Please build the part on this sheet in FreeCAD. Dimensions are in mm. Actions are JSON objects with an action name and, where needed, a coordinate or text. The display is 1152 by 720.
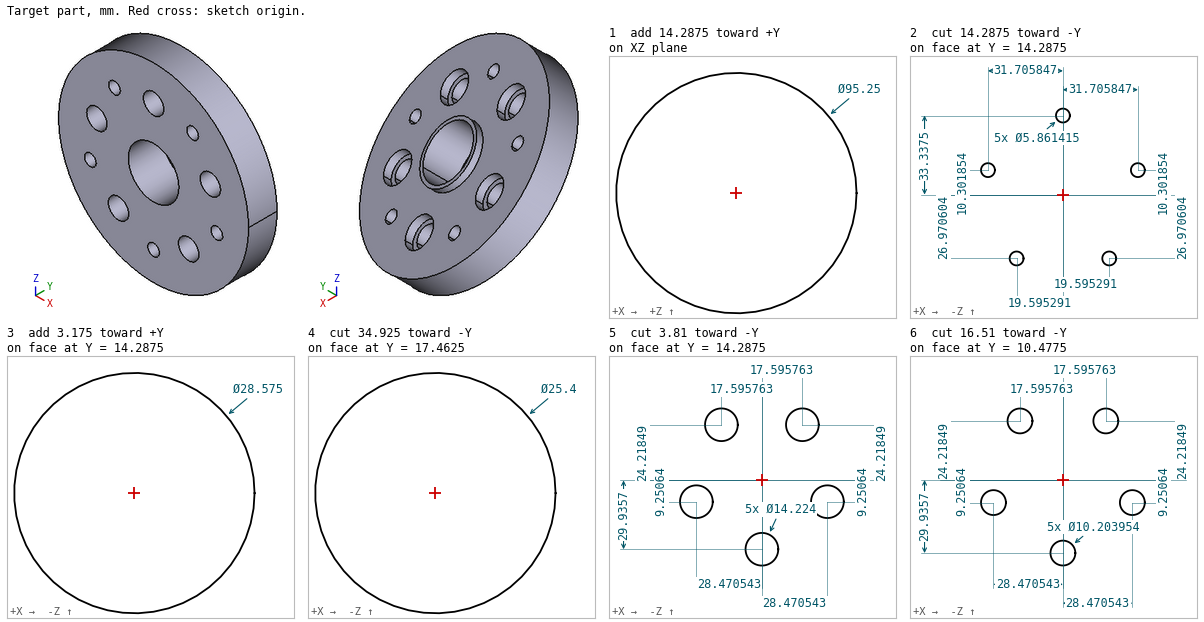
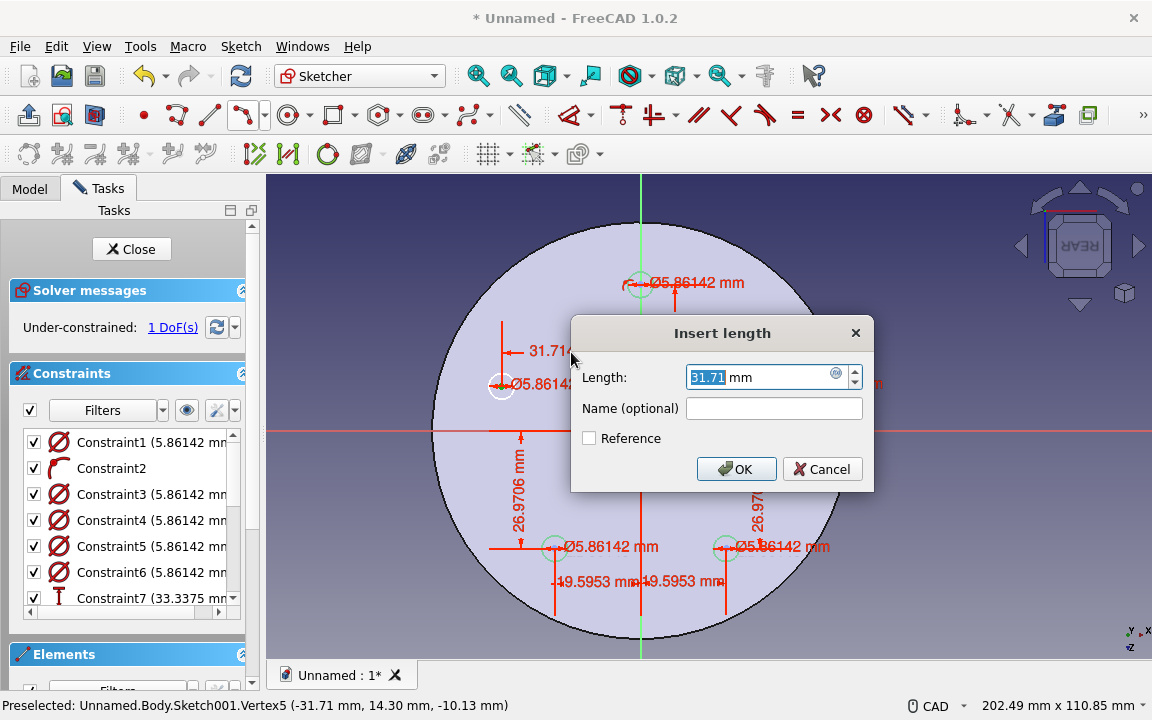
{"action": "type", "text": "31.705847"}
{"action": "key", "text": "Return"}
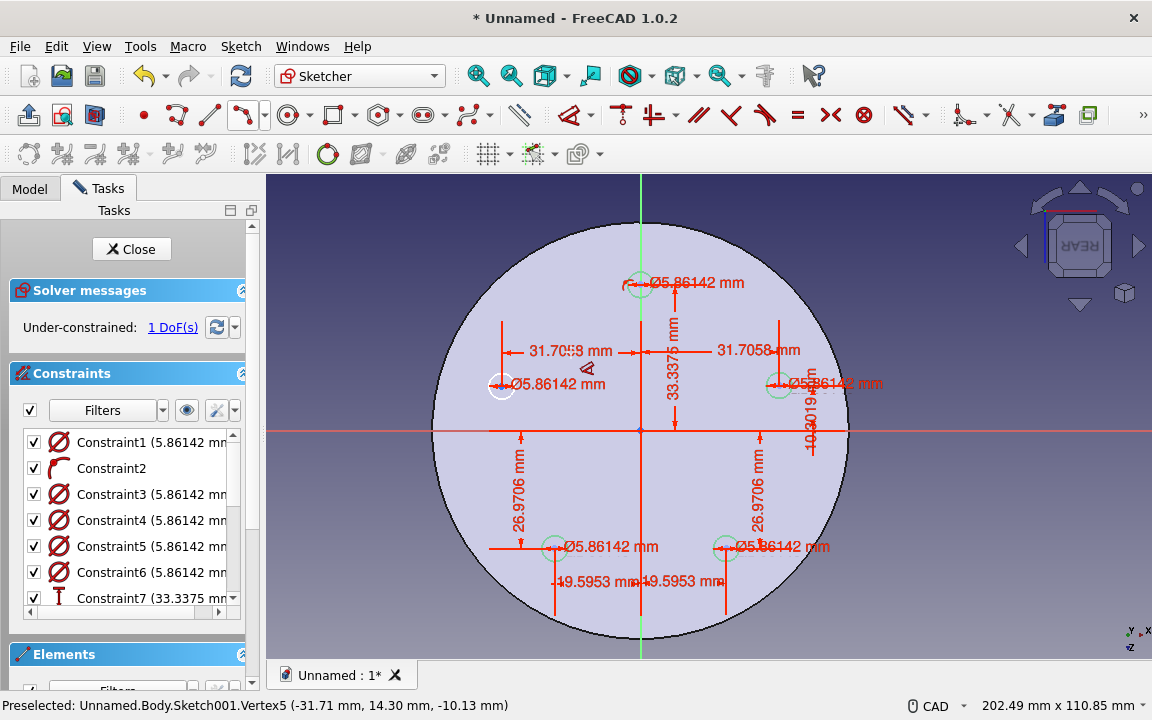
{"action": "left_click", "coordinate": [502, 386]}
{"action": "left_click", "coordinate": [468, 409]}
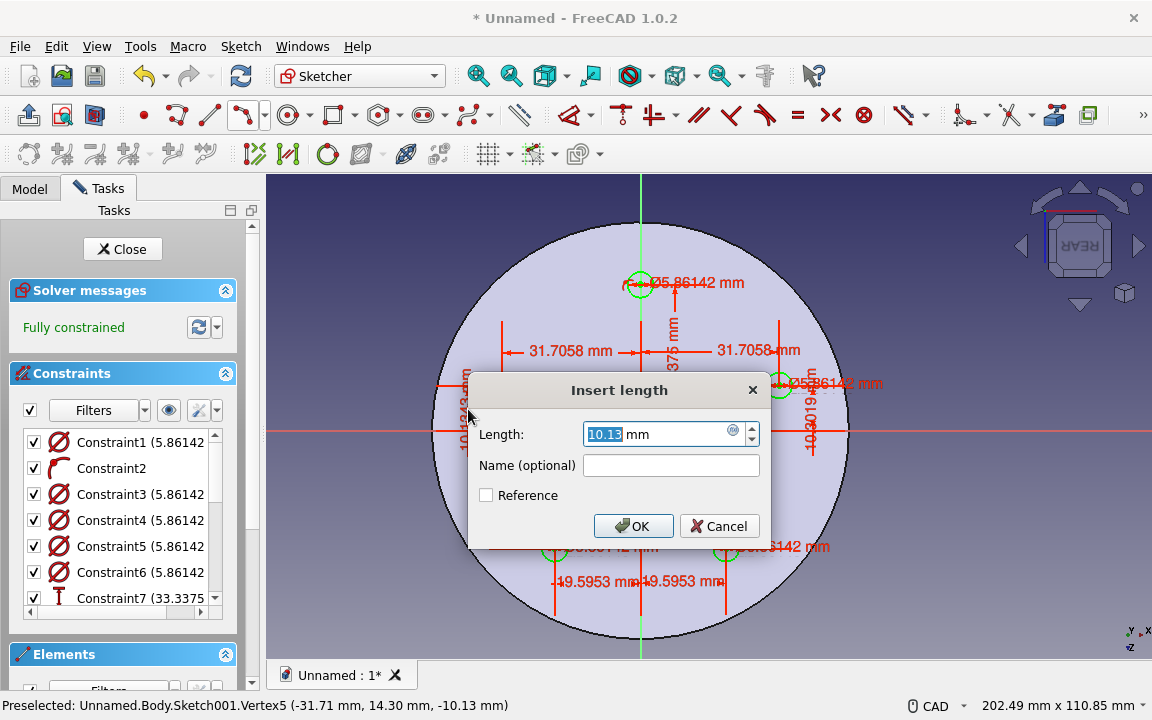
{"action": "type", "text": "10.301854"}
{"action": "key", "text": "Return"}
{"action": "key", "text": "Escape"}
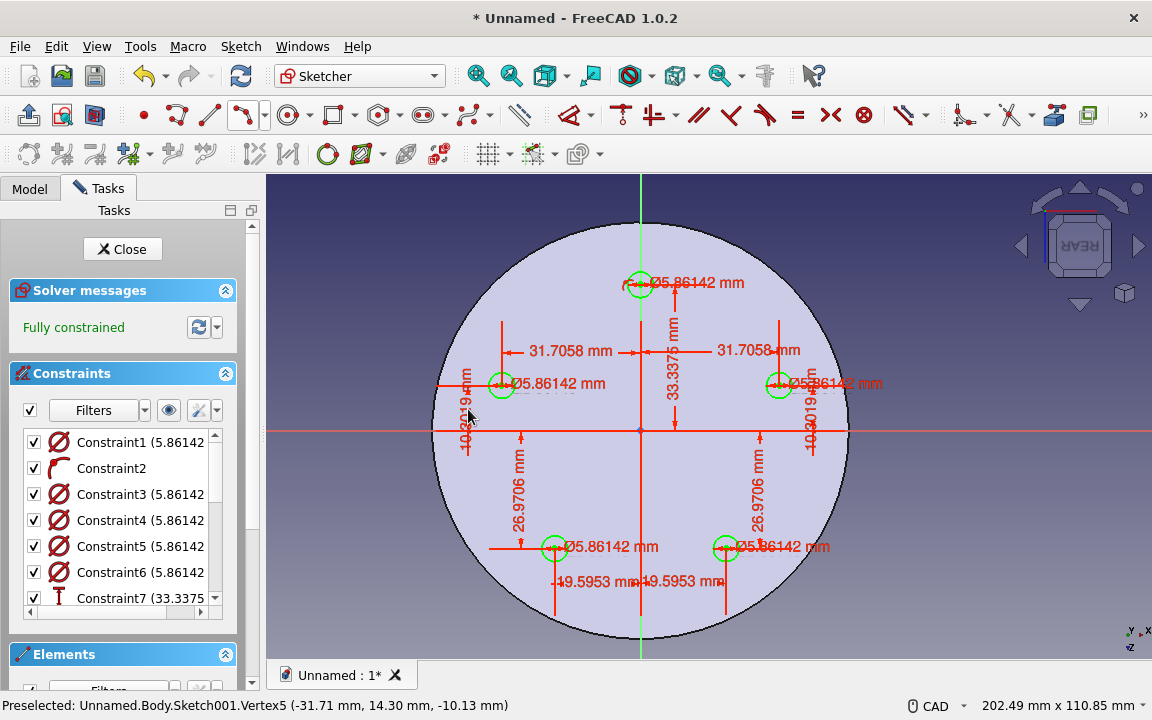
{"action": "left_click", "coordinate": [123, 249]}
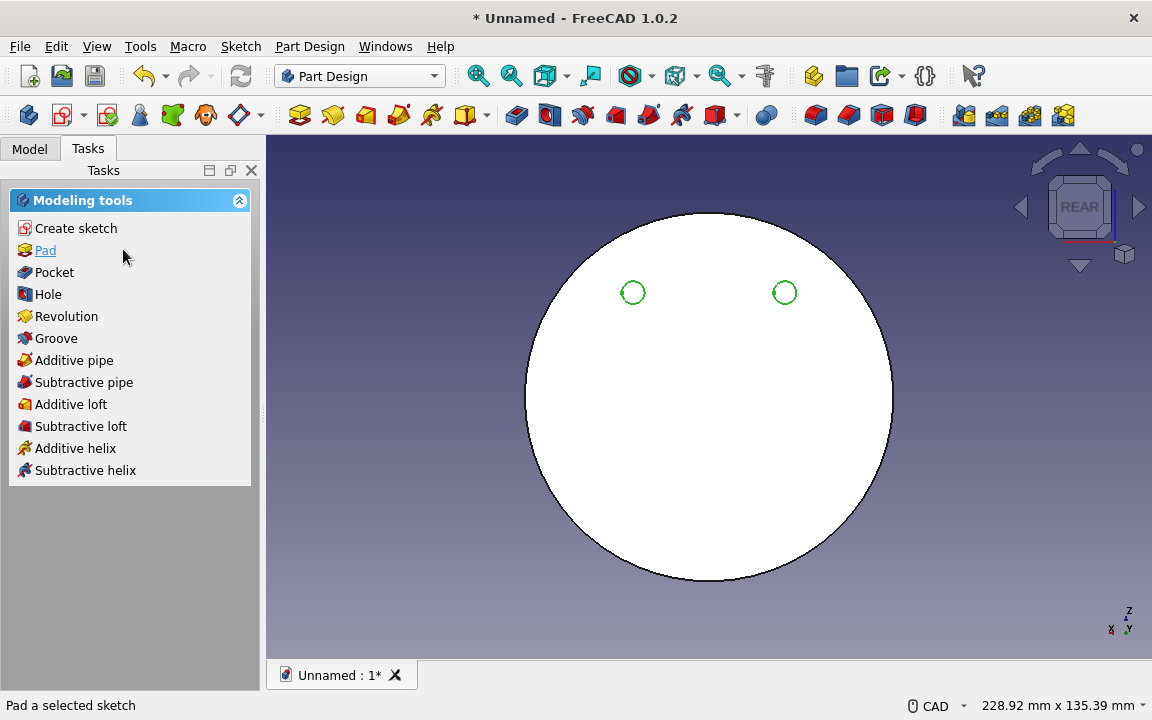
{"action": "left_click", "coordinate": [517, 116]}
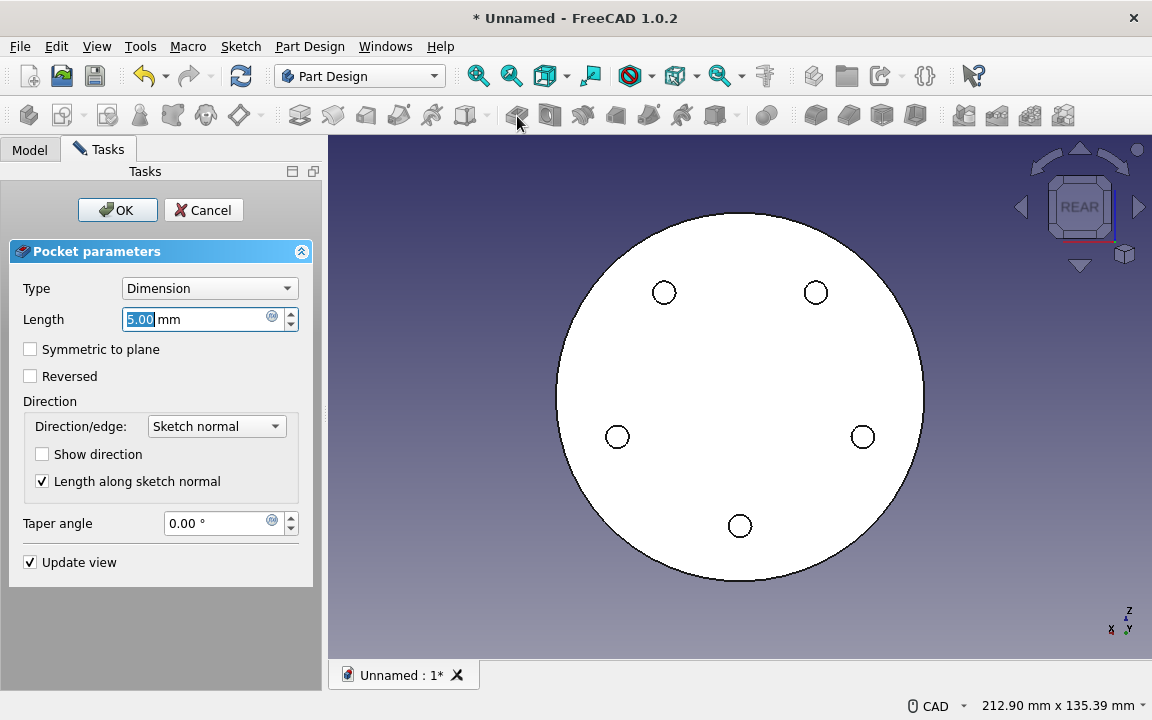
{"action": "type", "text": "14.2875"}
{"action": "key", "text": "Tab"}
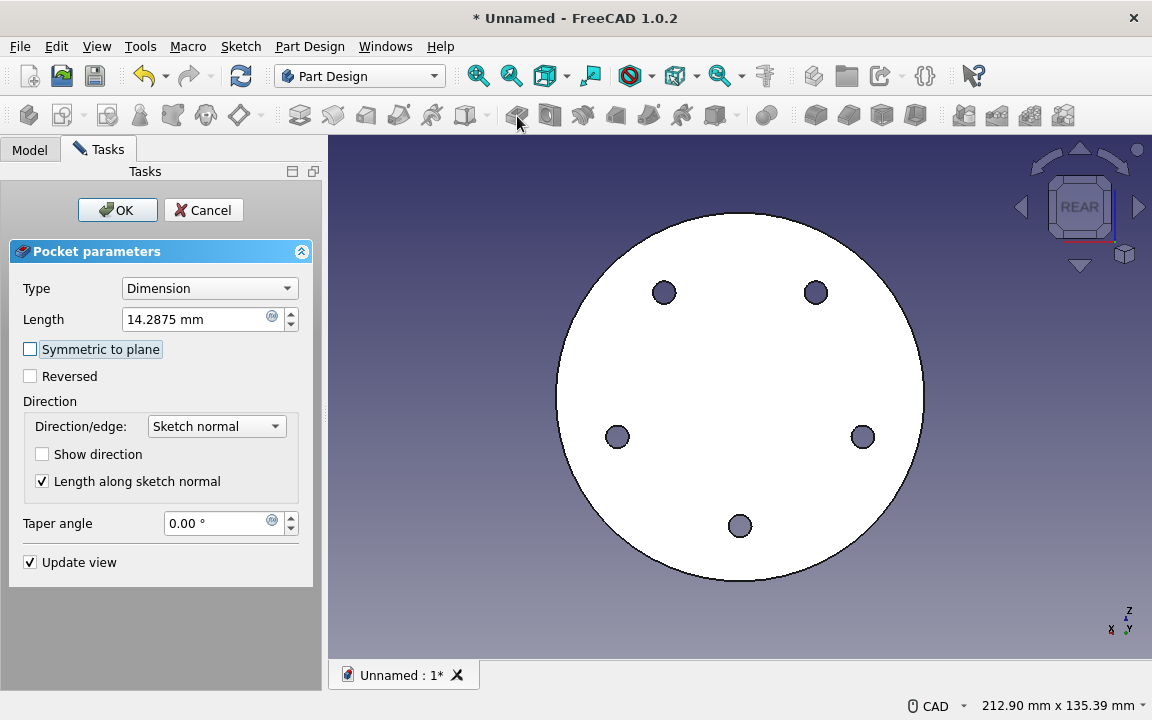
{"action": "left_click", "coordinate": [118, 210]}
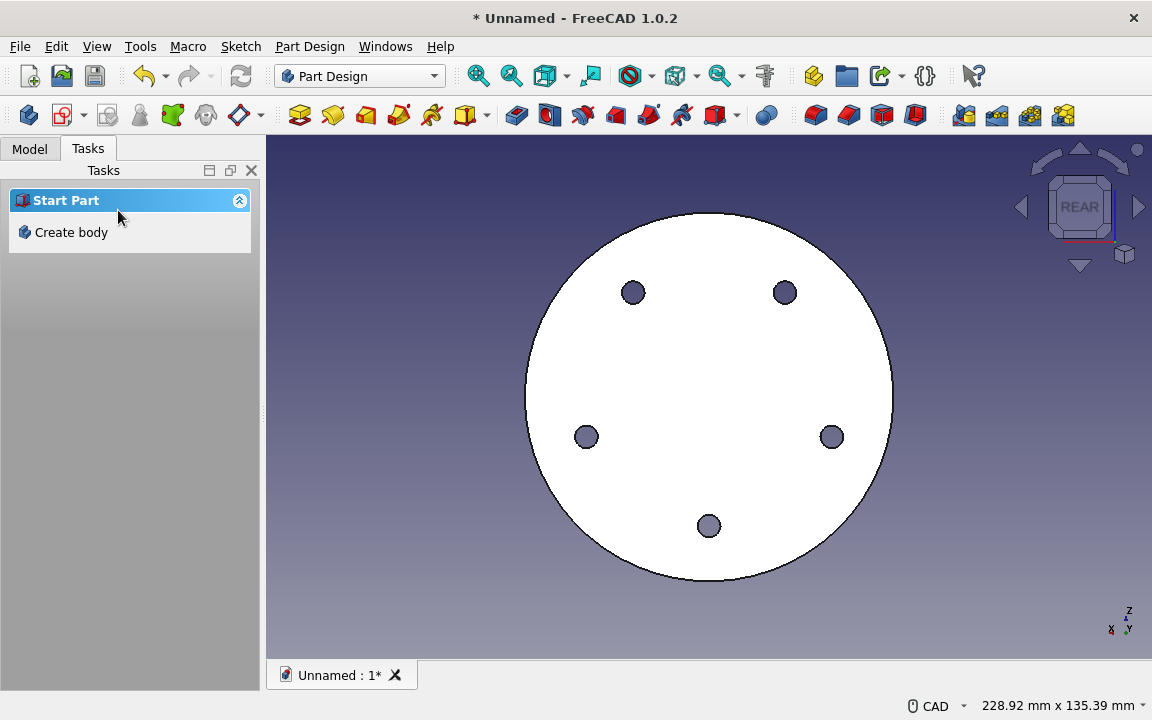
{"action": "left_click", "coordinate": [709, 396]}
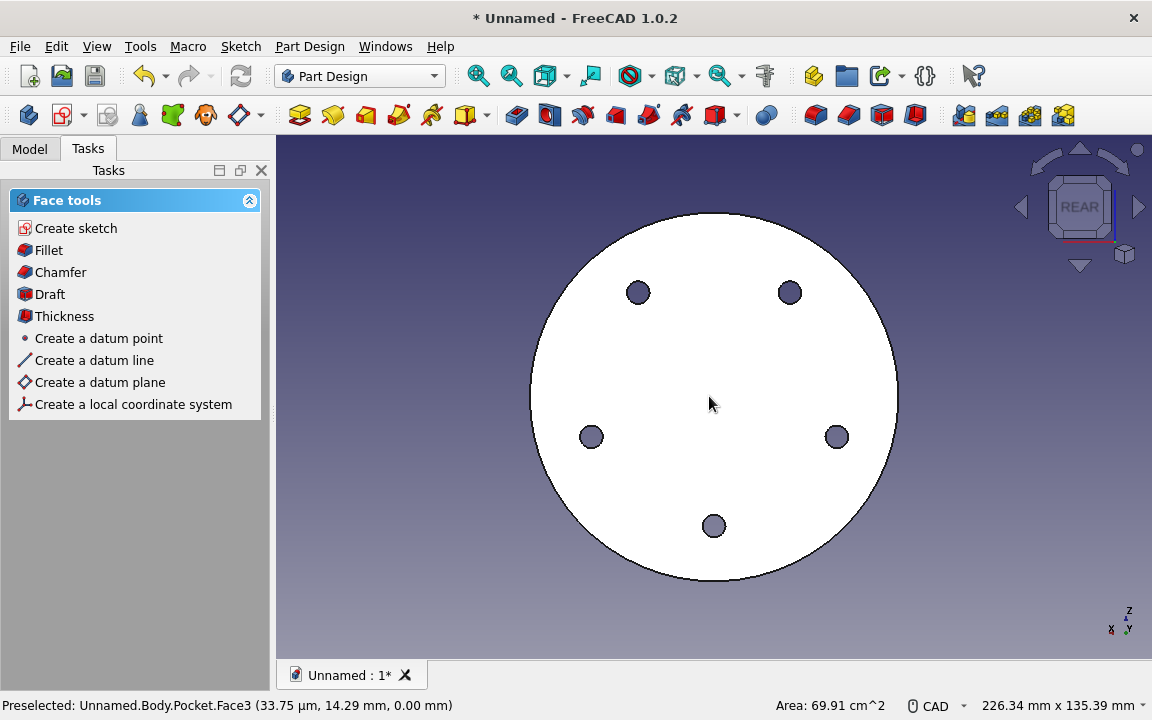
{"action": "left_click", "coordinate": [62, 116]}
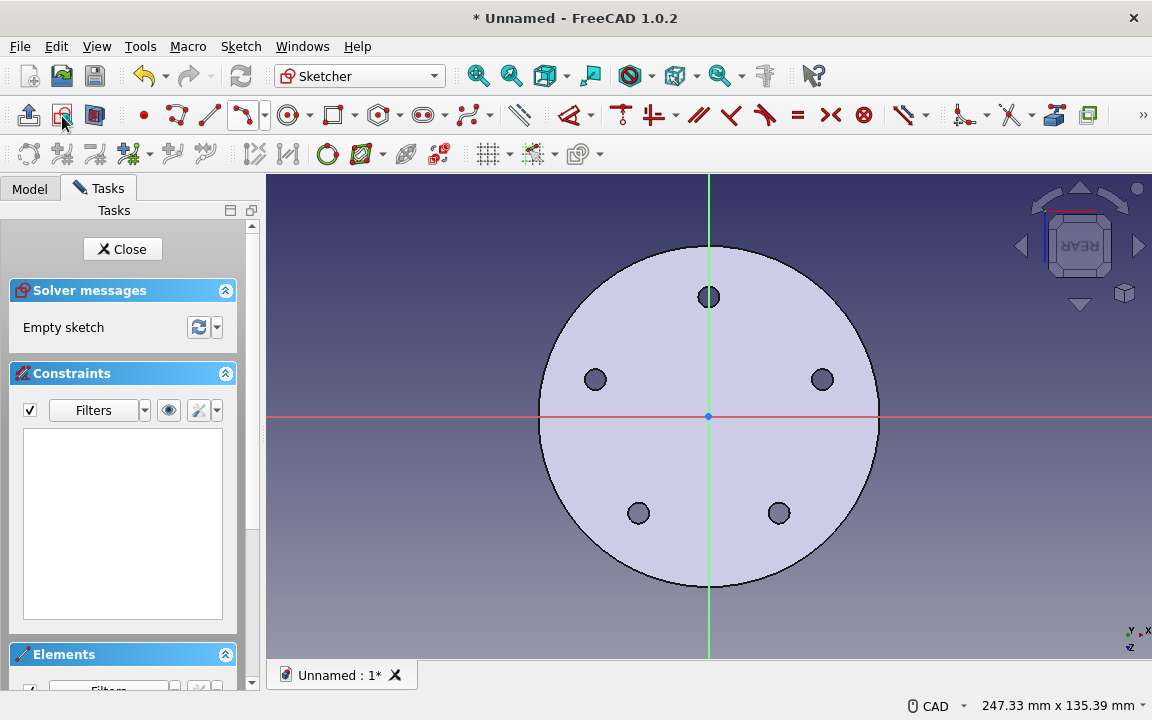
{"action": "scroll", "coordinate": [749, 416], "scroll_direction": "up", "scroll_amount": 5}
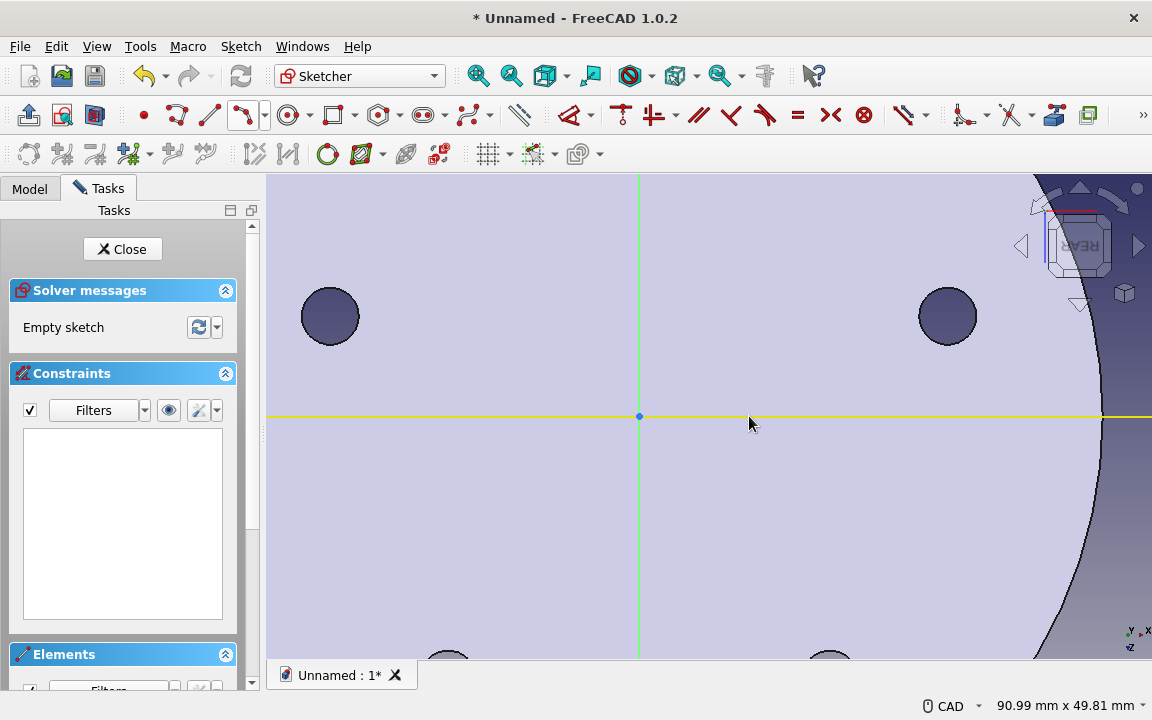
{"action": "left_click", "coordinate": [288, 116]}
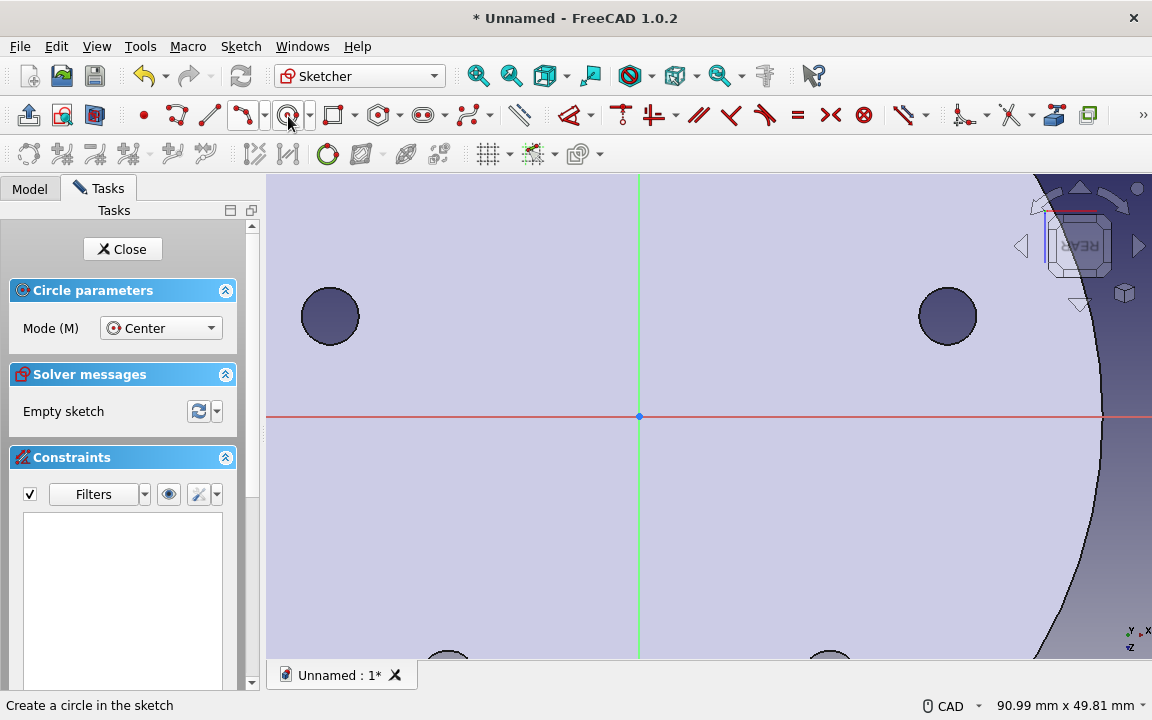
{"action": "left_click", "coordinate": [639, 416]}
{"action": "mouse_move", "coordinate": [737, 318]}